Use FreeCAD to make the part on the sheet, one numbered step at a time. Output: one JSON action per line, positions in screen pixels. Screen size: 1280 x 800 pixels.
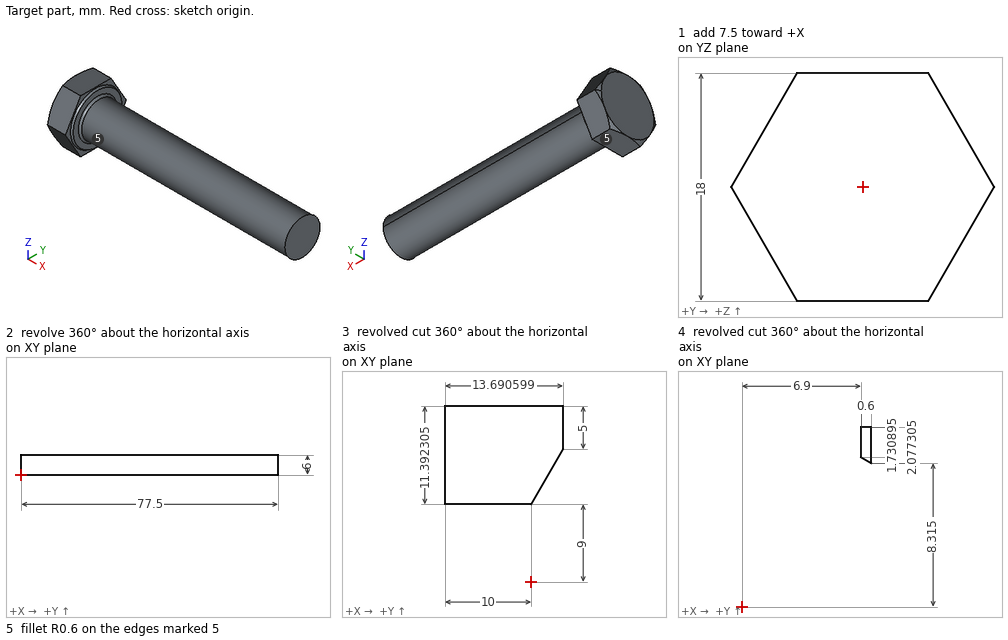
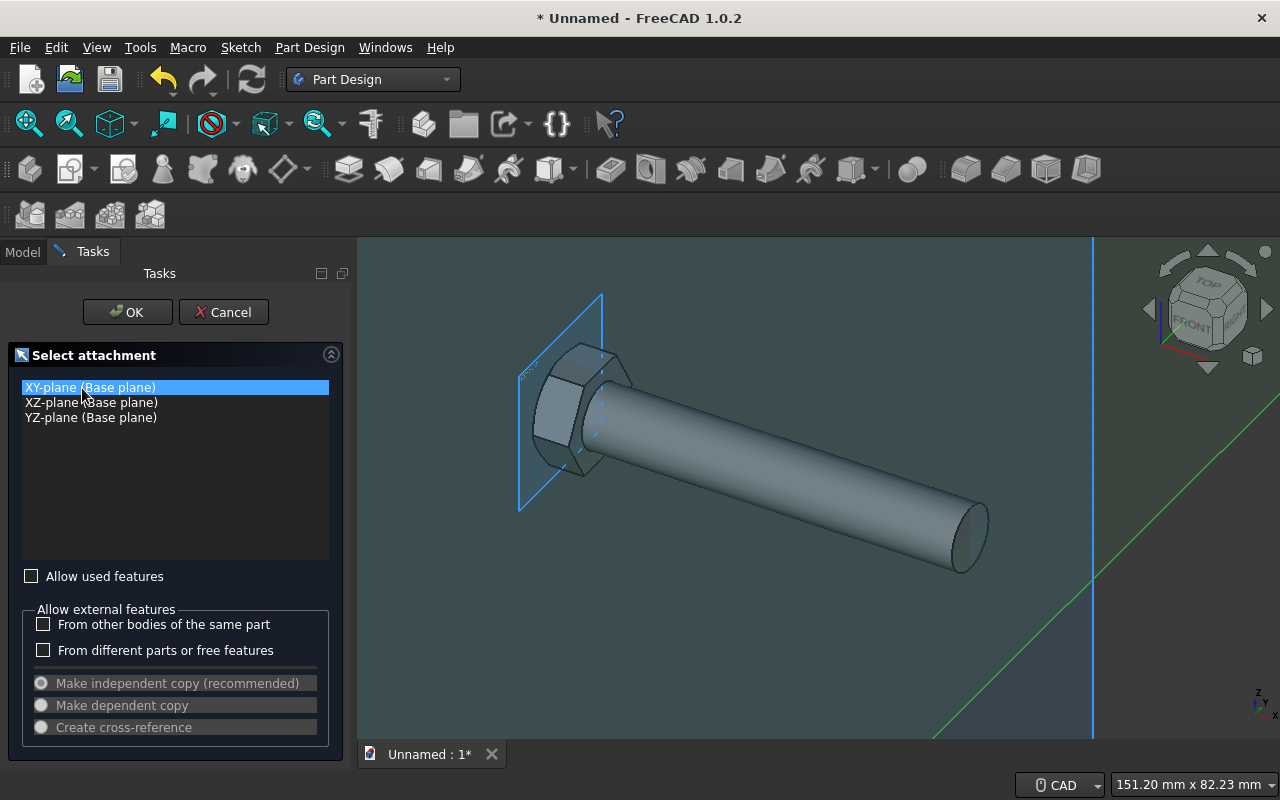
{"action": "left_click", "coordinate": [128, 312]}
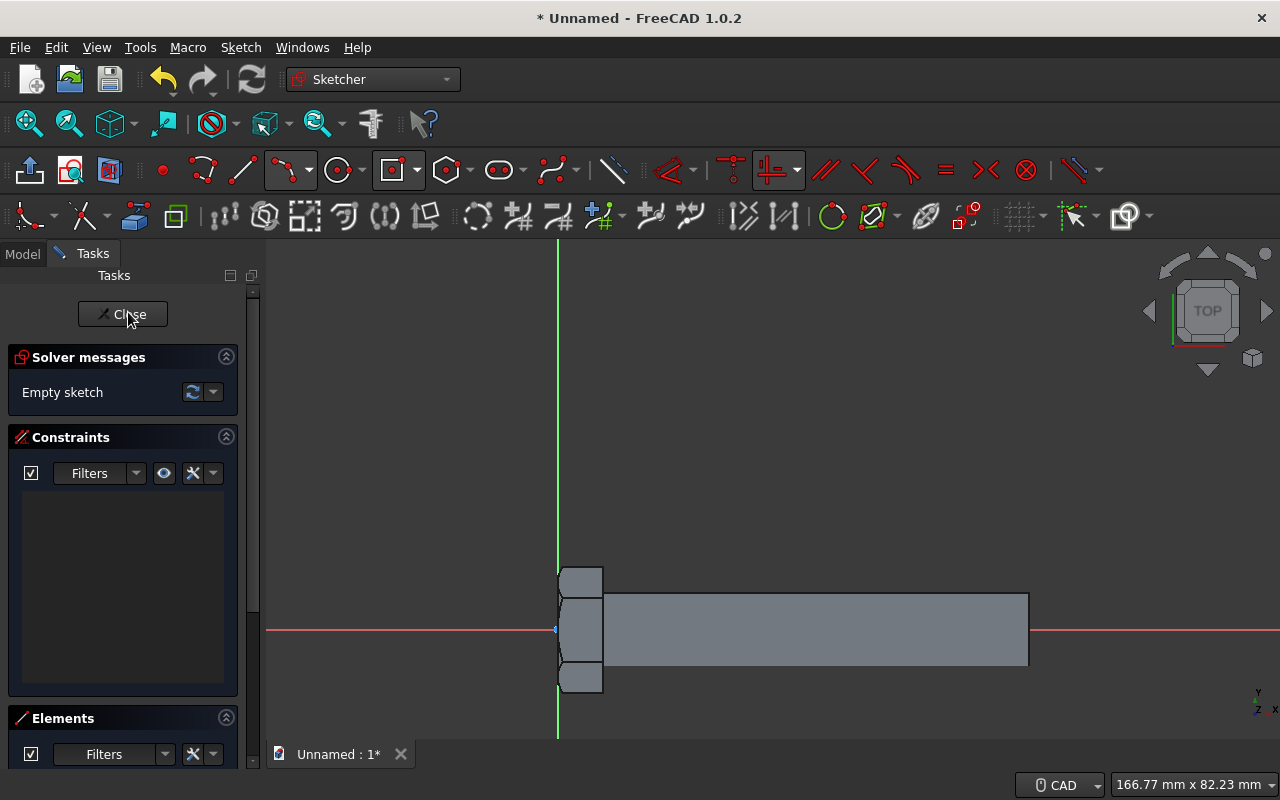
{"action": "left_click", "coordinate": [110, 170]}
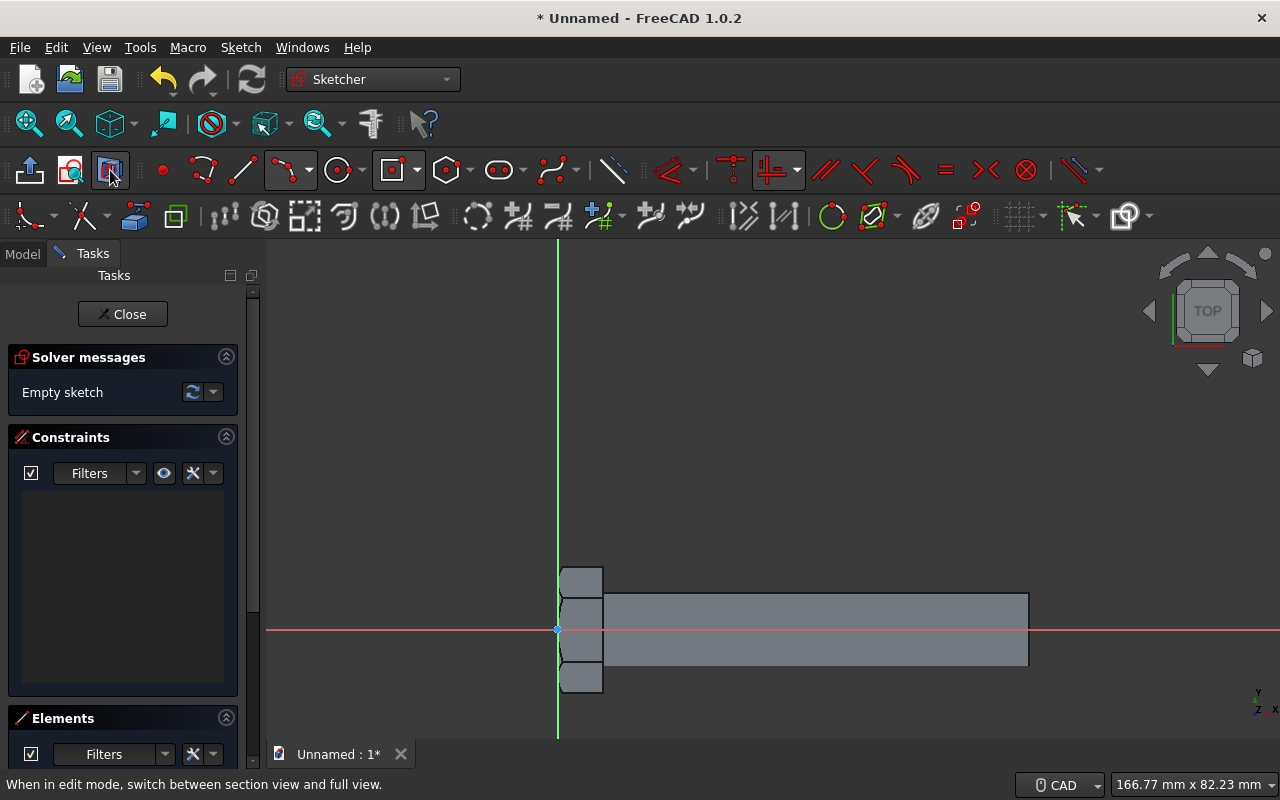
{"action": "scroll", "coordinate": [596, 577], "scroll_direction": "up", "scroll_amount": 15}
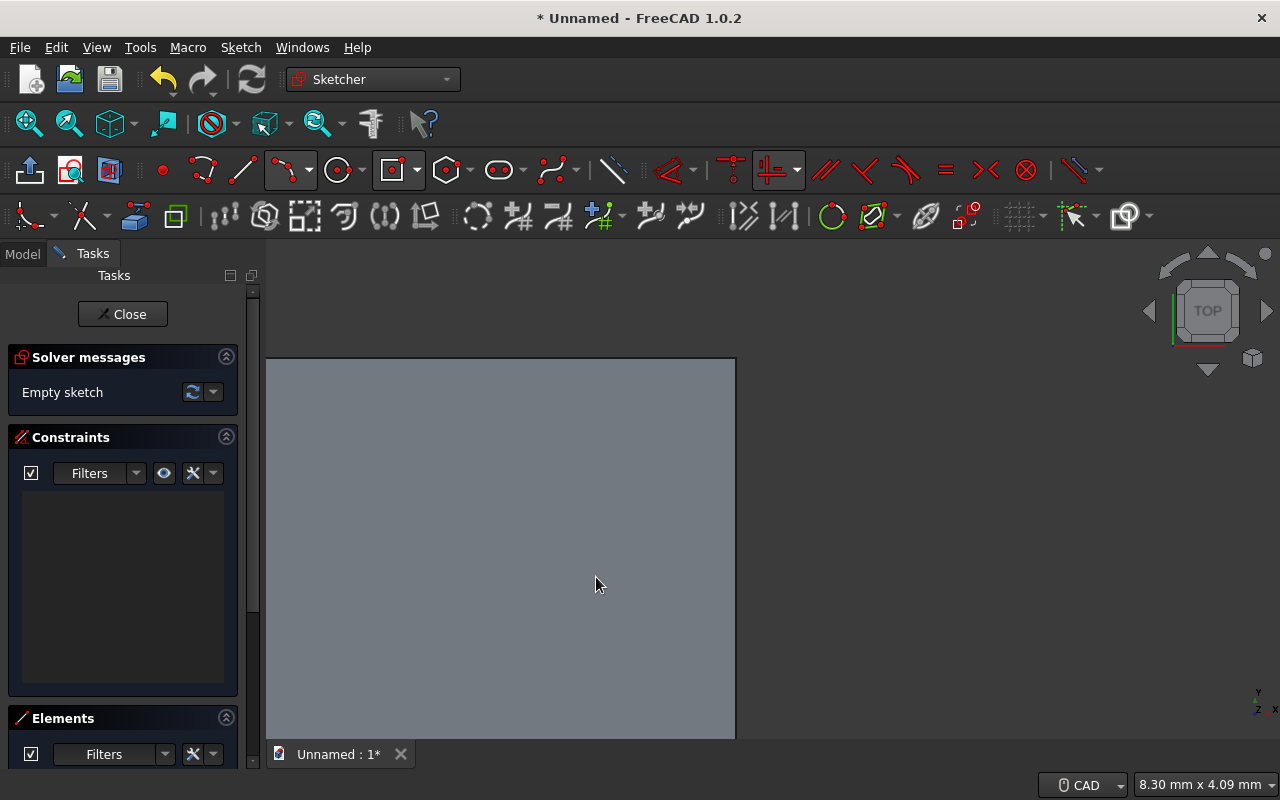
{"action": "left_click", "coordinate": [204, 170]}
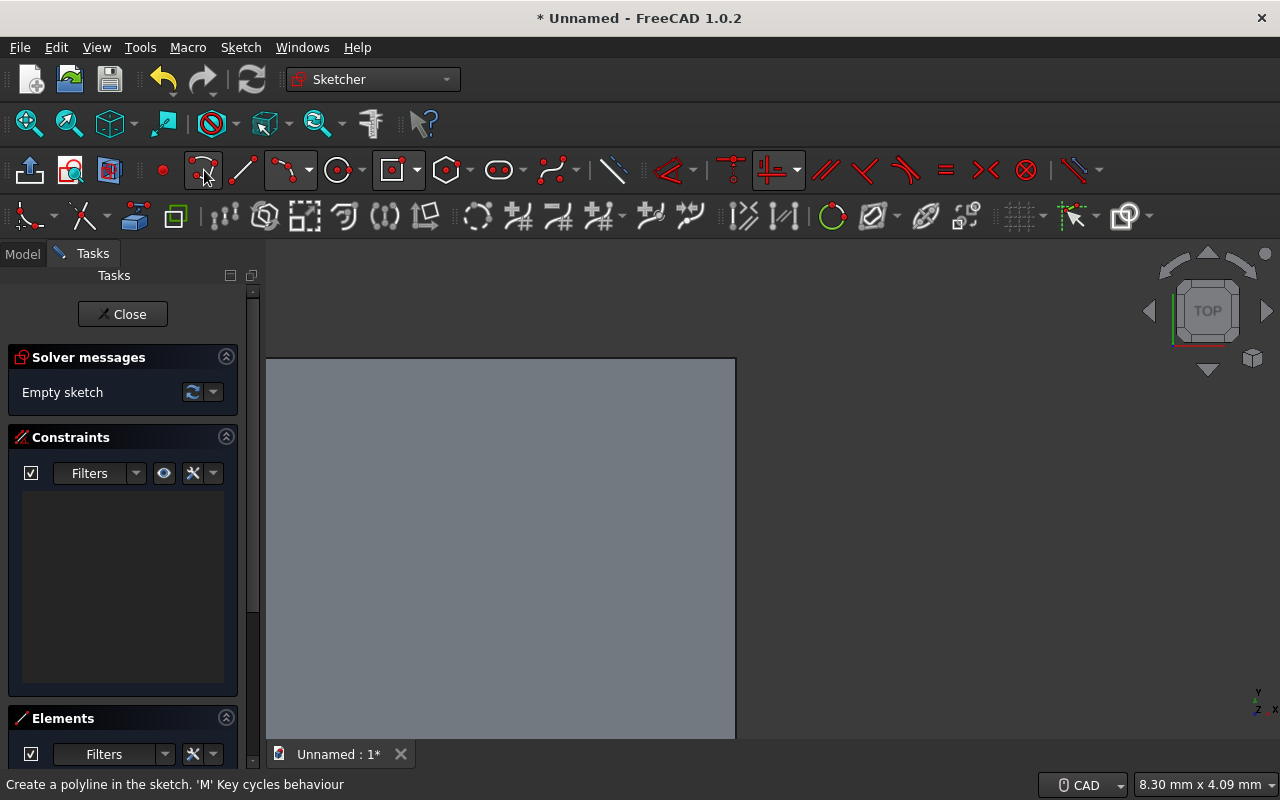
{"action": "left_click", "coordinate": [663, 569]}
{"action": "left_click", "coordinate": [736, 611]}
{"action": "left_click", "coordinate": [736, 358]}
{"action": "left_click", "coordinate": [663, 358]}
{"action": "left_click", "coordinate": [663, 570]}
{"action": "key", "text": "Escape"}
{"action": "key", "text": "Escape"}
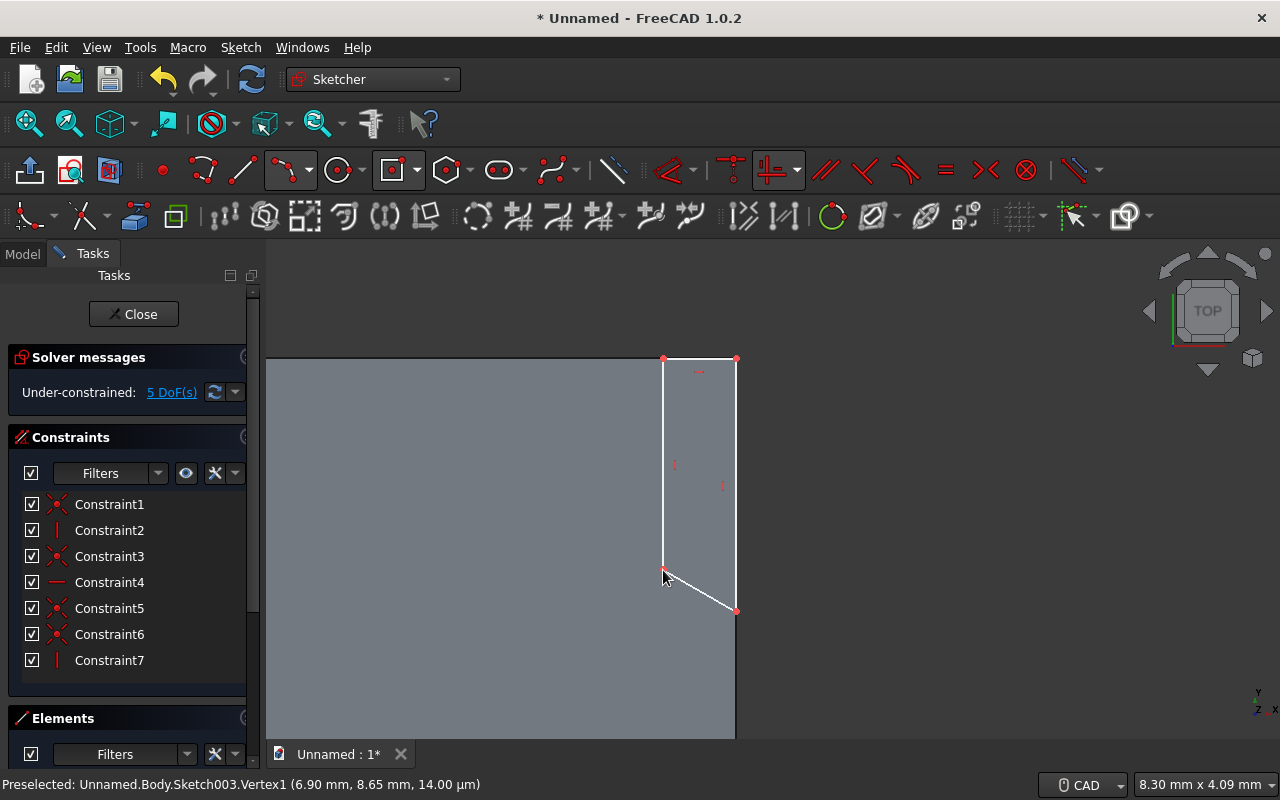
{"action": "left_click", "coordinate": [668, 170]}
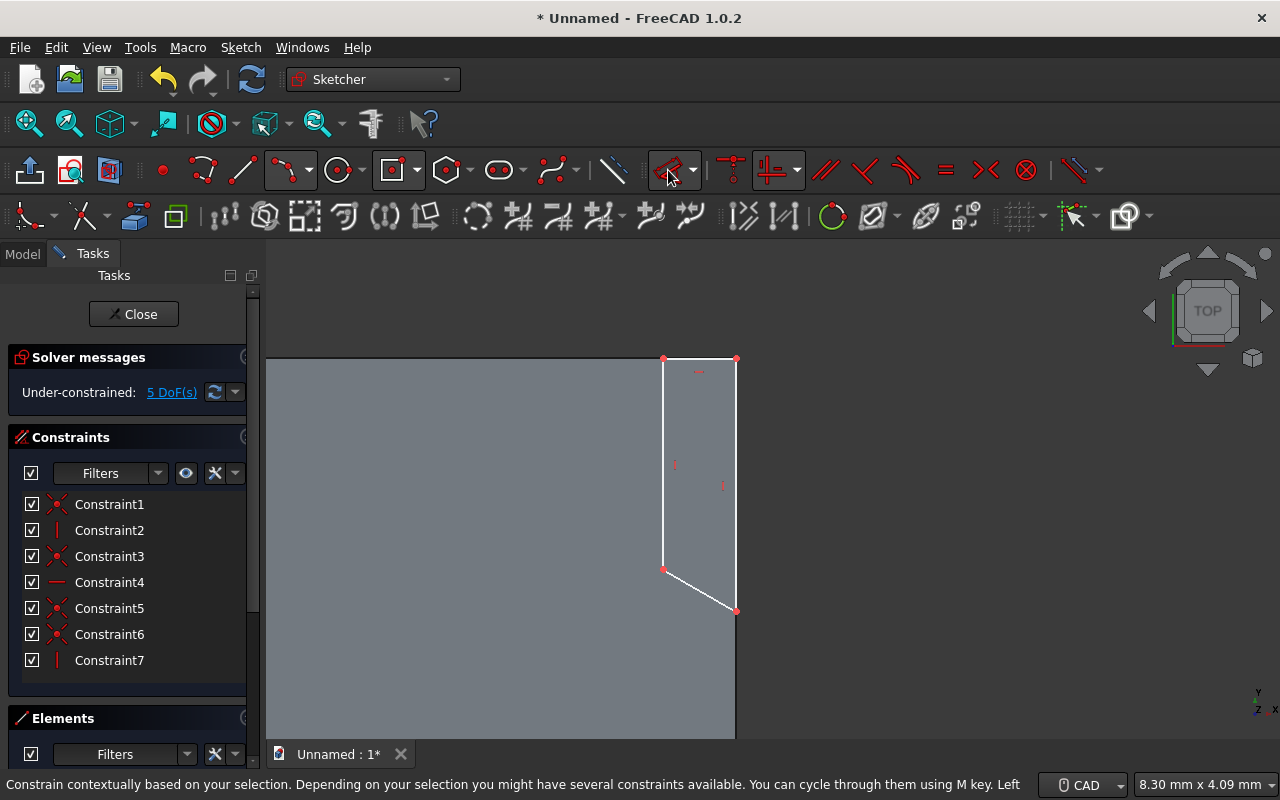
{"action": "left_click", "coordinate": [714, 359]}
{"action": "left_click", "coordinate": [699, 325]}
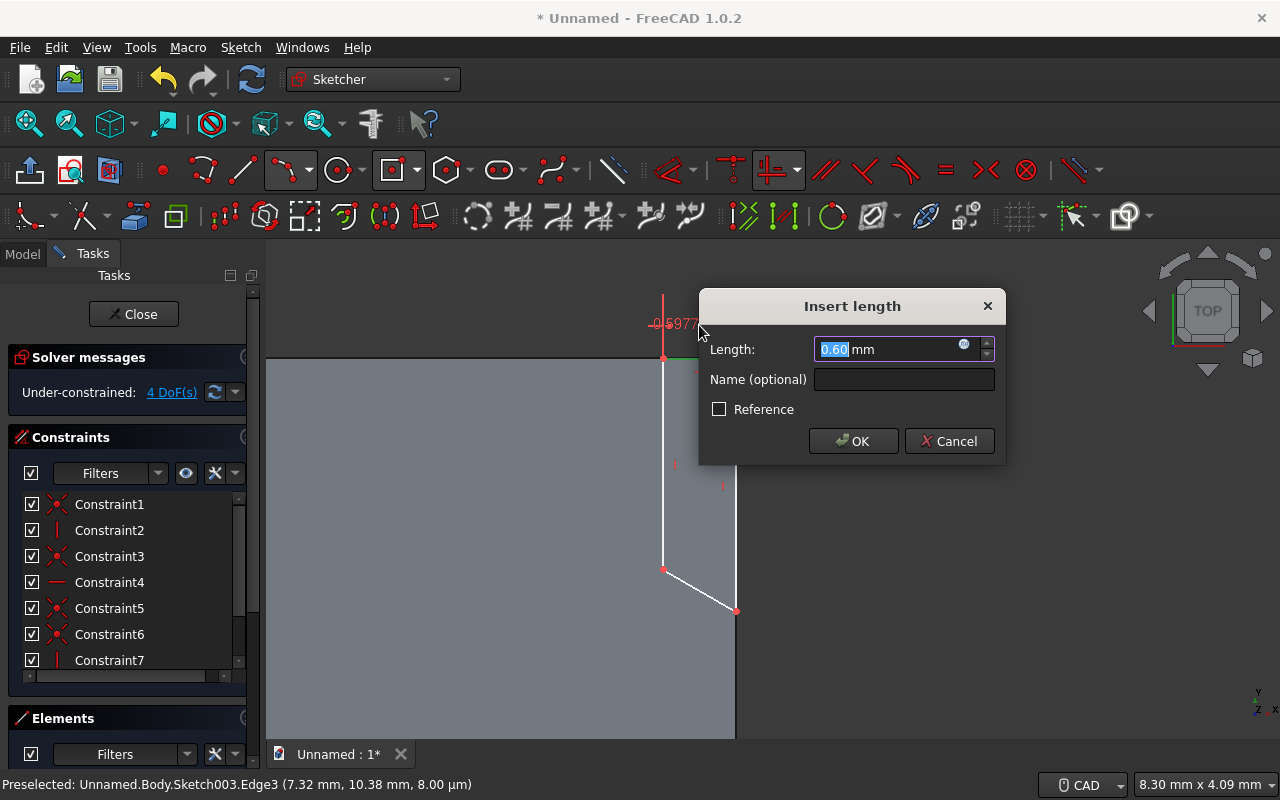
{"action": "type", "text": "0.6"}
{"action": "key", "text": "Return"}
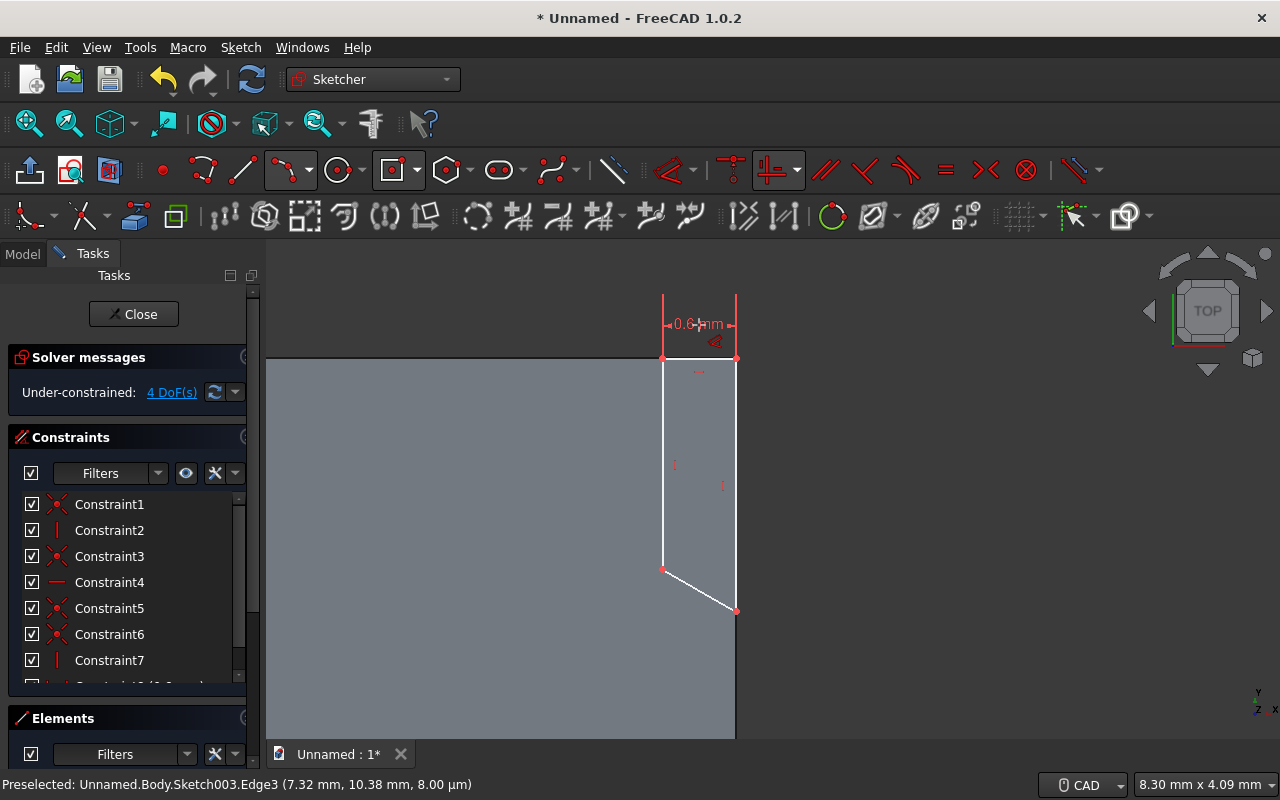
{"action": "left_click", "coordinate": [663, 570]}
{"action": "left_click", "coordinate": [478, 536]}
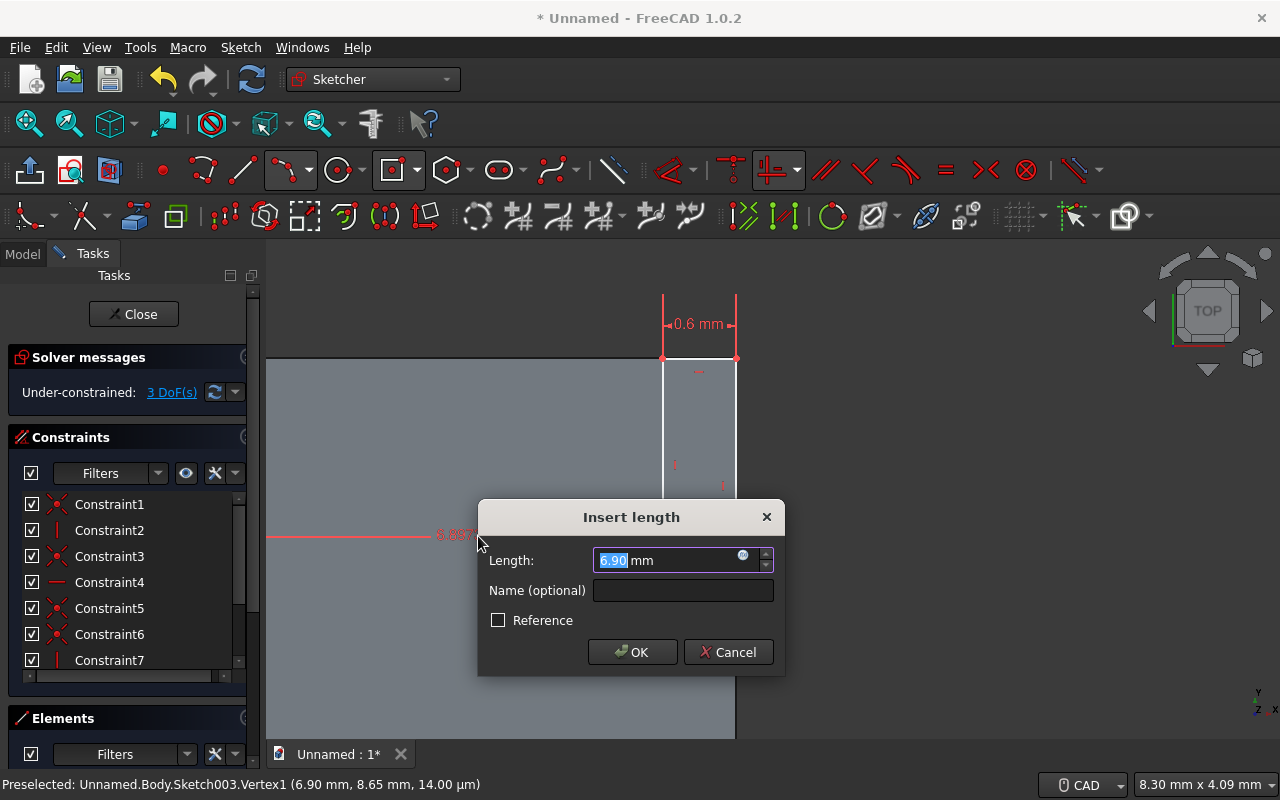
{"action": "type", "text": "6.9"}
{"action": "key", "text": "Return"}